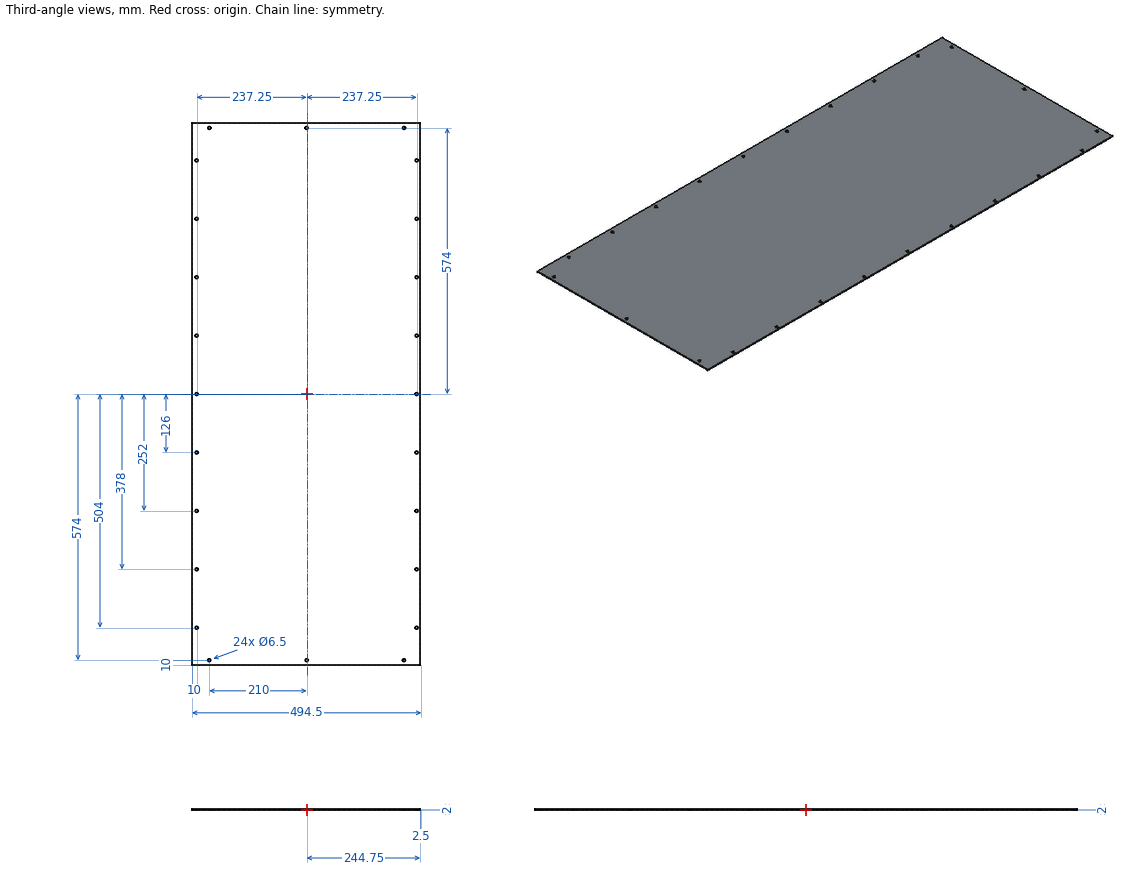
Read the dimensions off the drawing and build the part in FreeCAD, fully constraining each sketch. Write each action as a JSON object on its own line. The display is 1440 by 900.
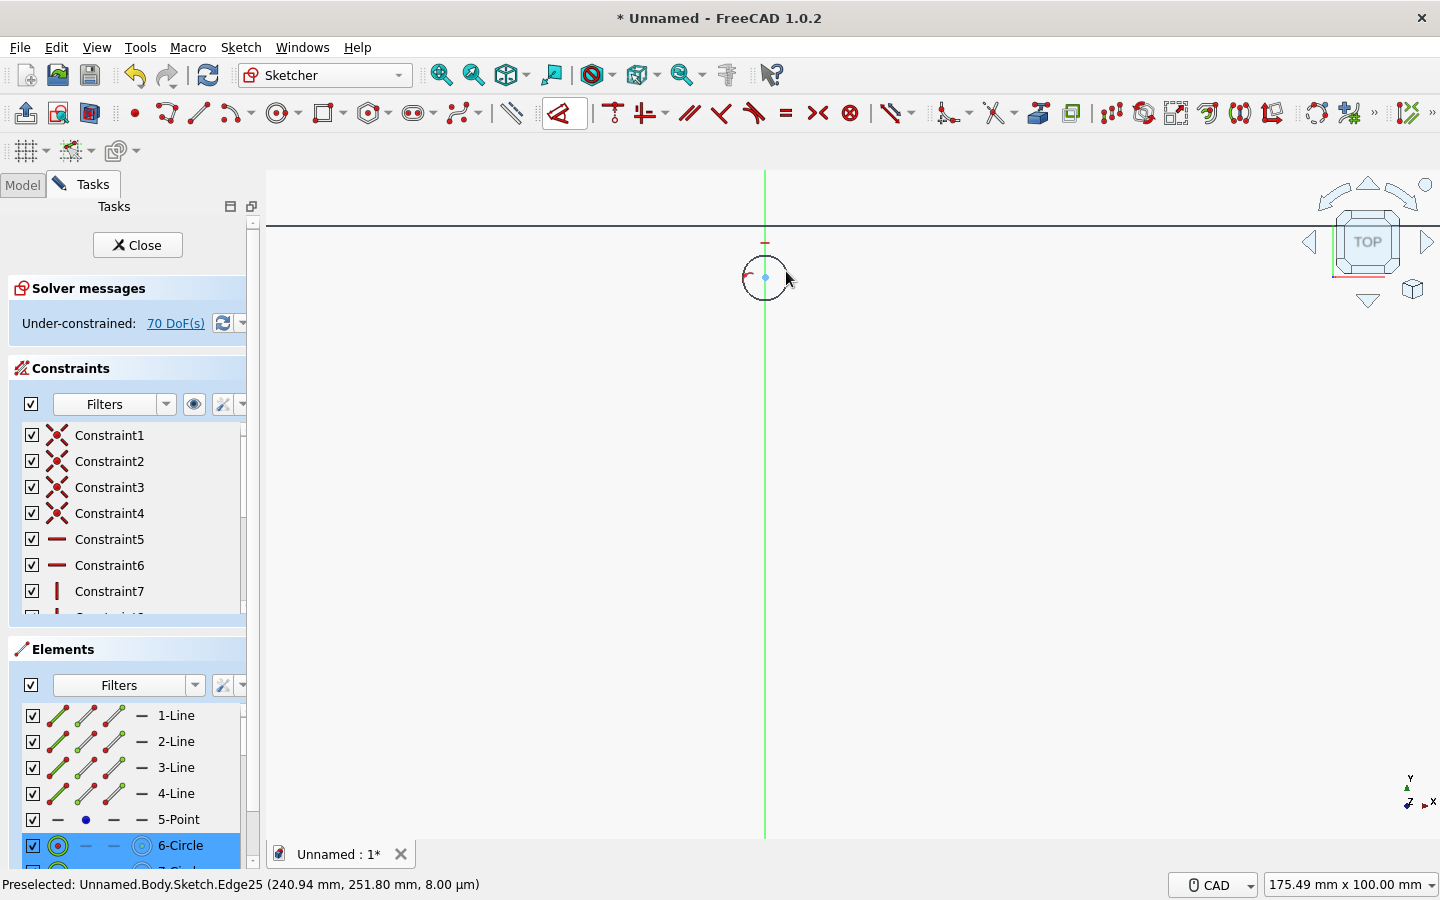
{"action": "left_click", "coordinate": [781, 262]}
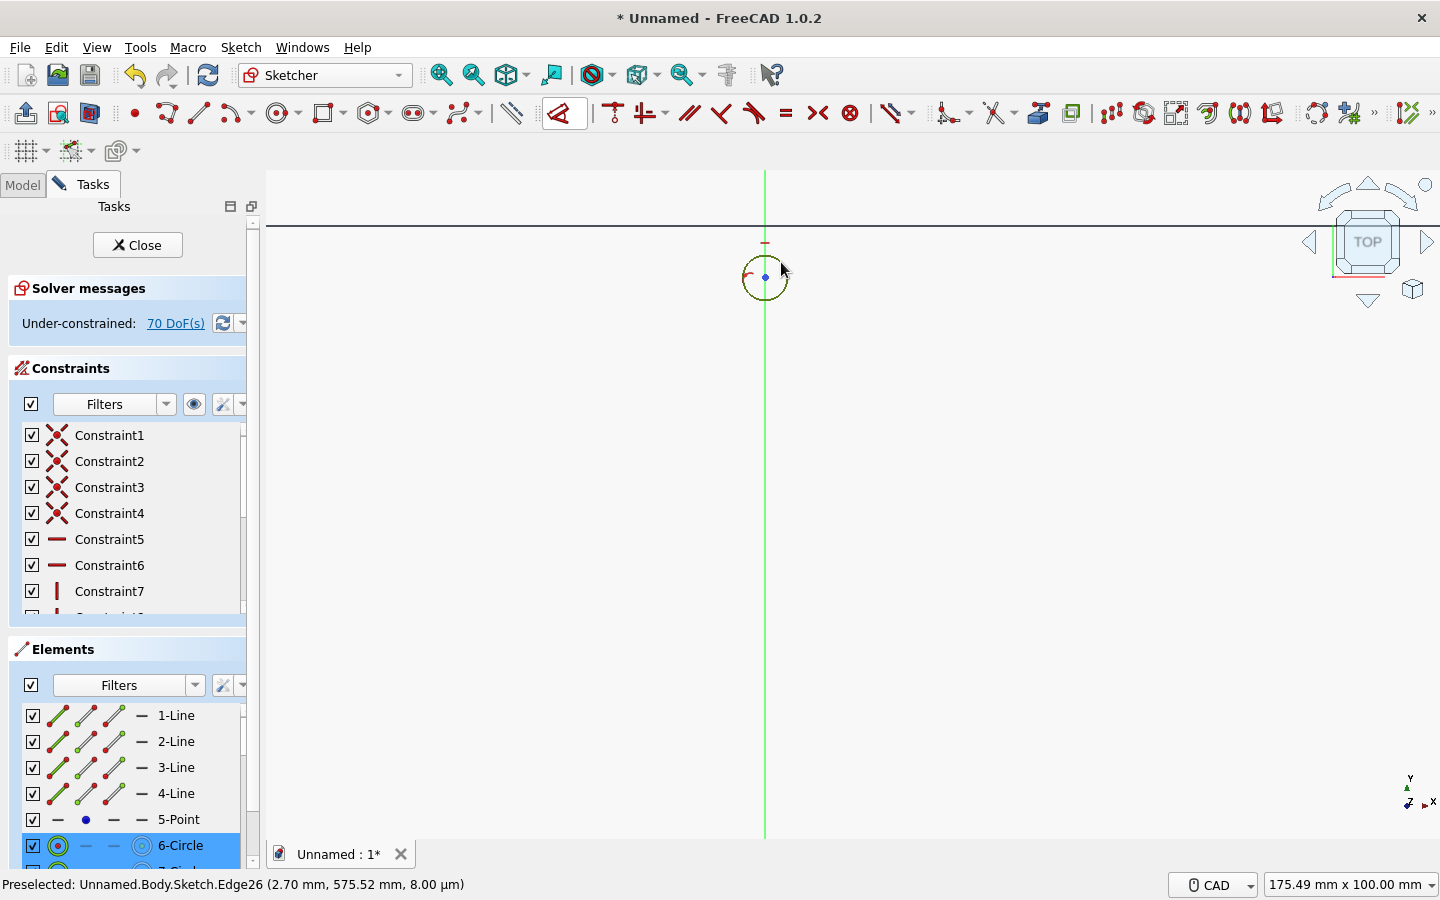
{"action": "scroll", "coordinate": [786, 271], "scroll_direction": "down", "scroll_amount": 14}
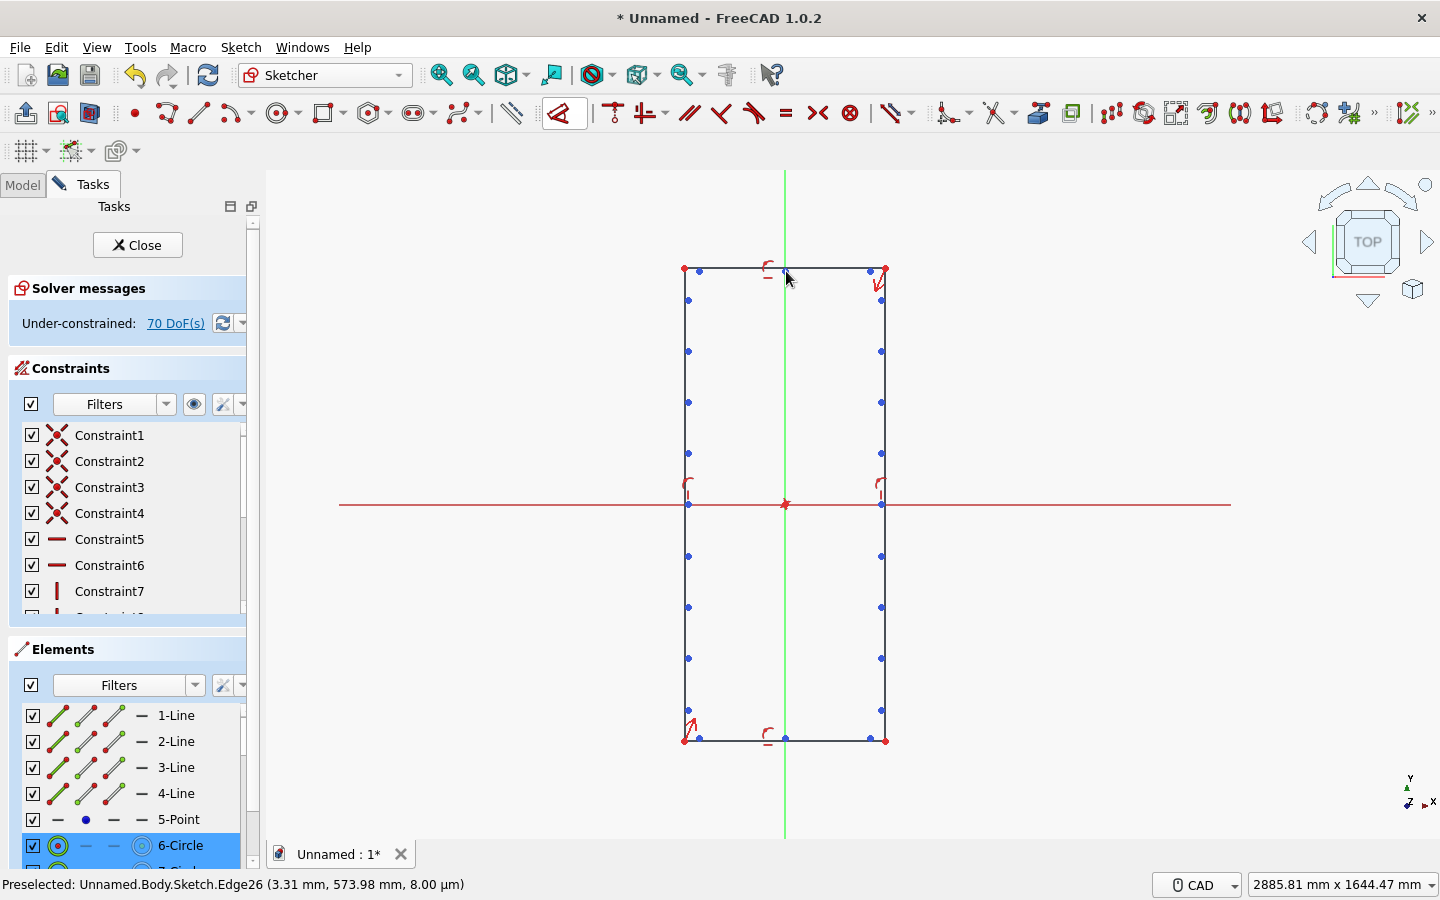
{"action": "scroll", "coordinate": [883, 350], "scroll_direction": "up", "scroll_amount": 12}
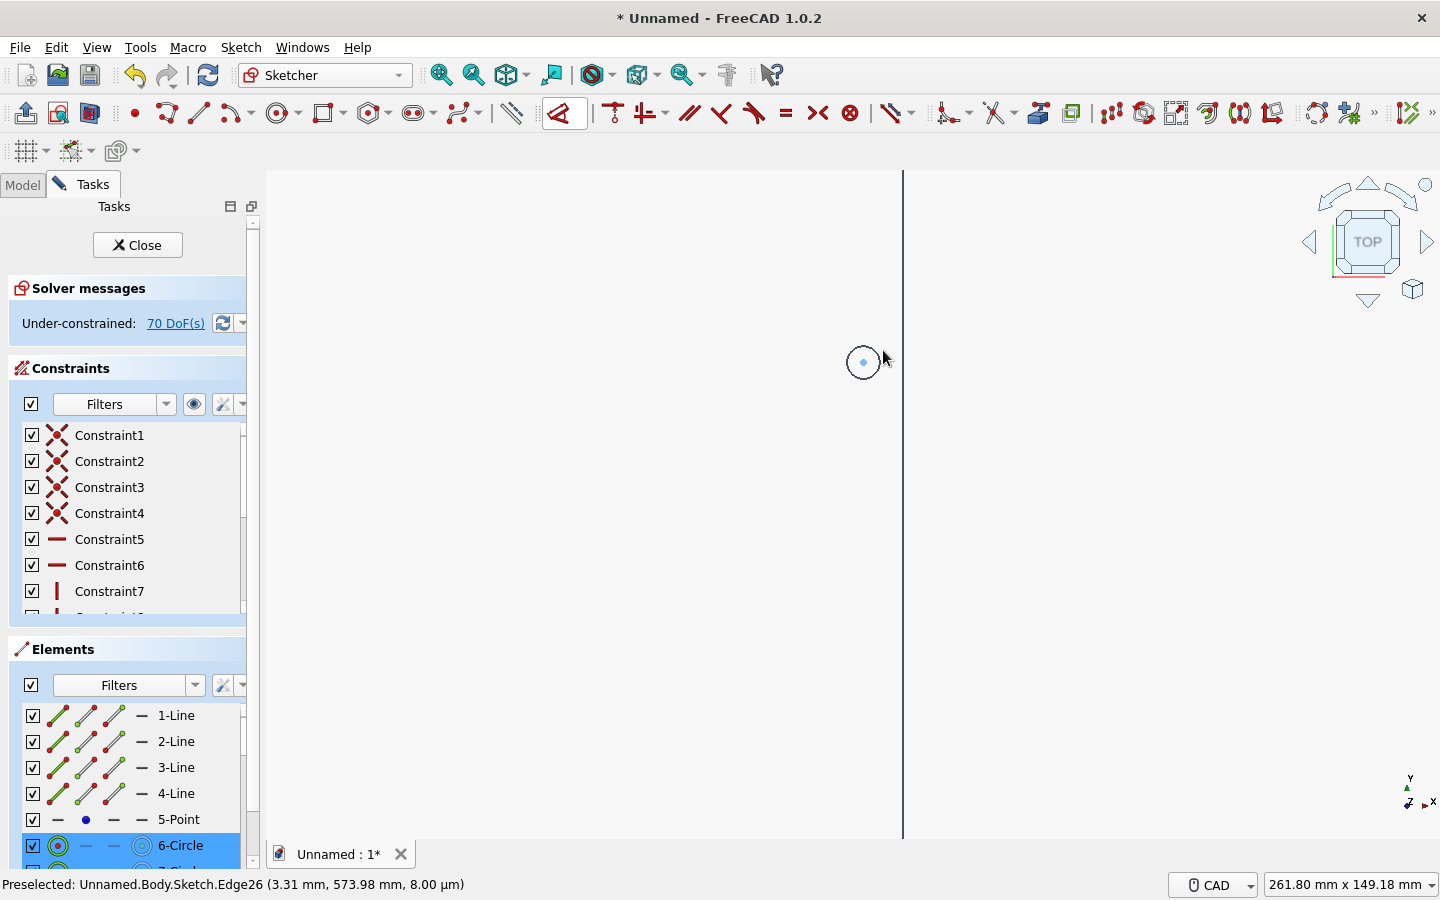
{"action": "left_click", "coordinate": [875, 351]}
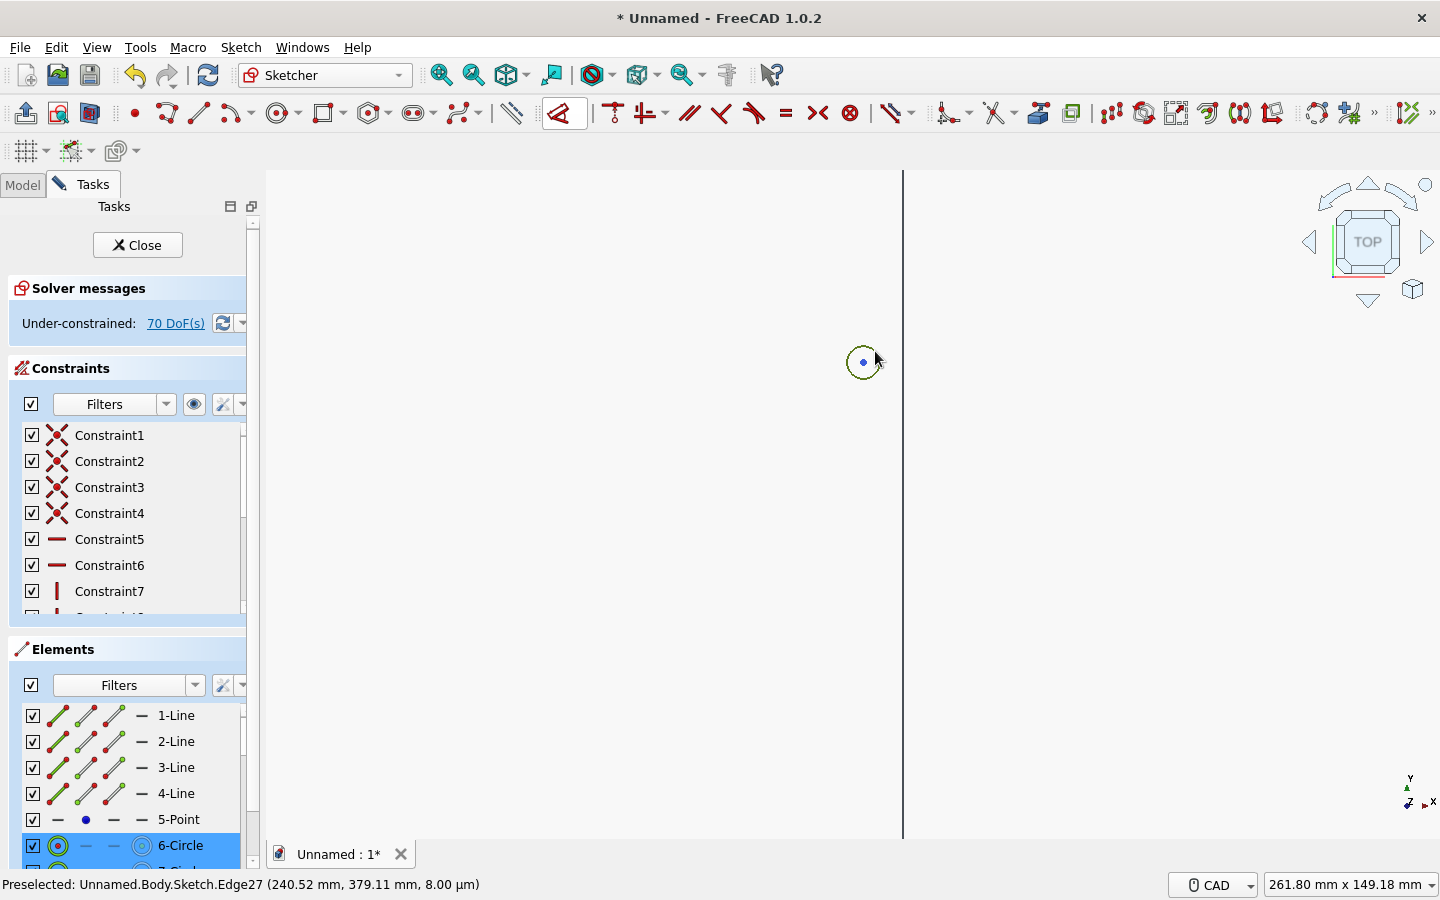
{"action": "scroll", "coordinate": [883, 350], "scroll_direction": "down", "scroll_amount": 12}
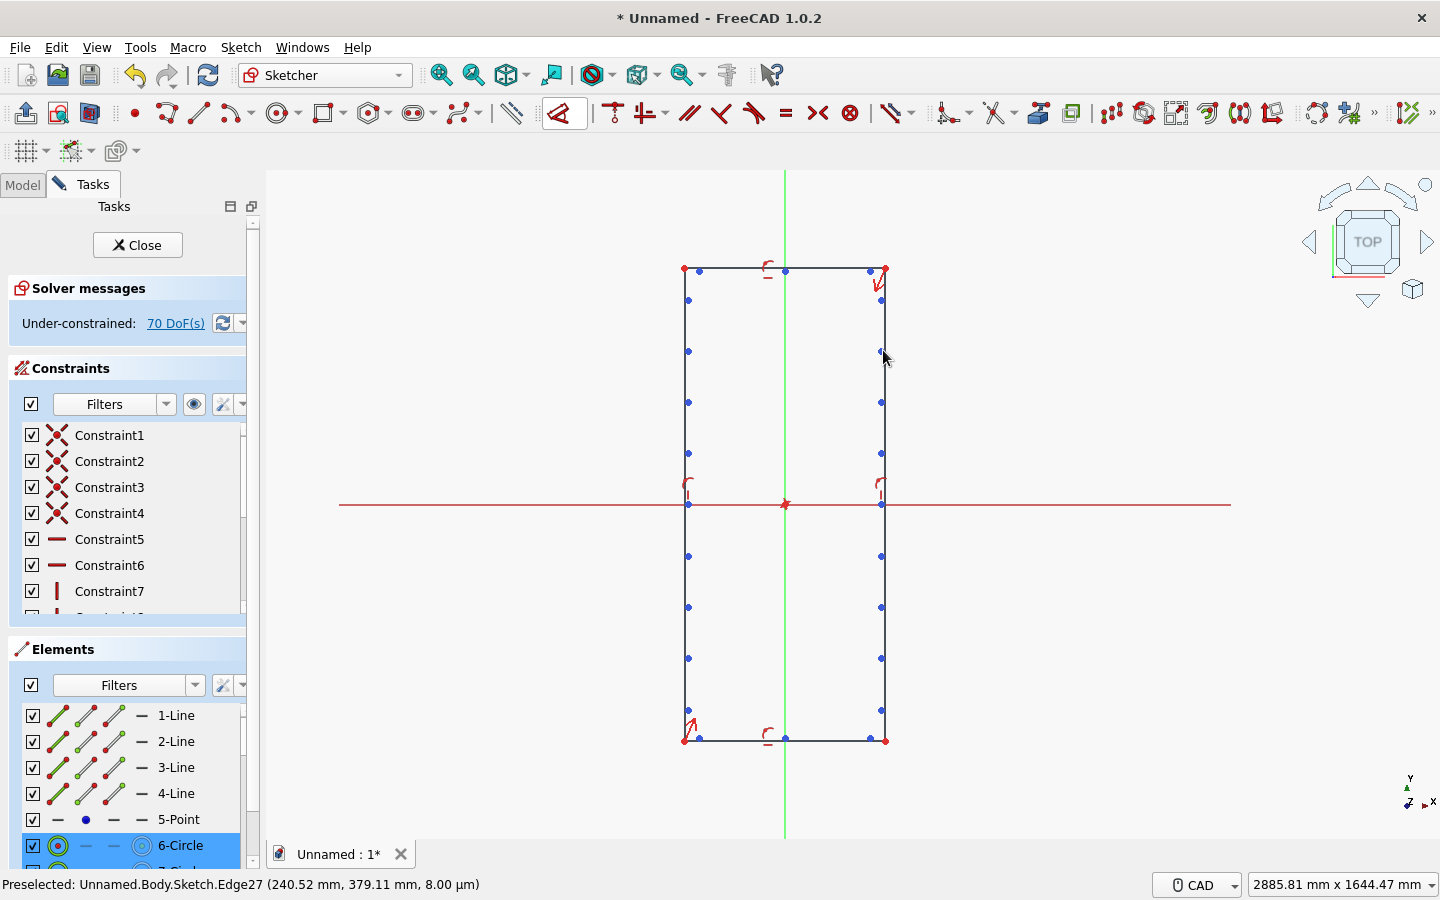
{"action": "scroll", "coordinate": [883, 299], "scroll_direction": "up", "scroll_amount": 12}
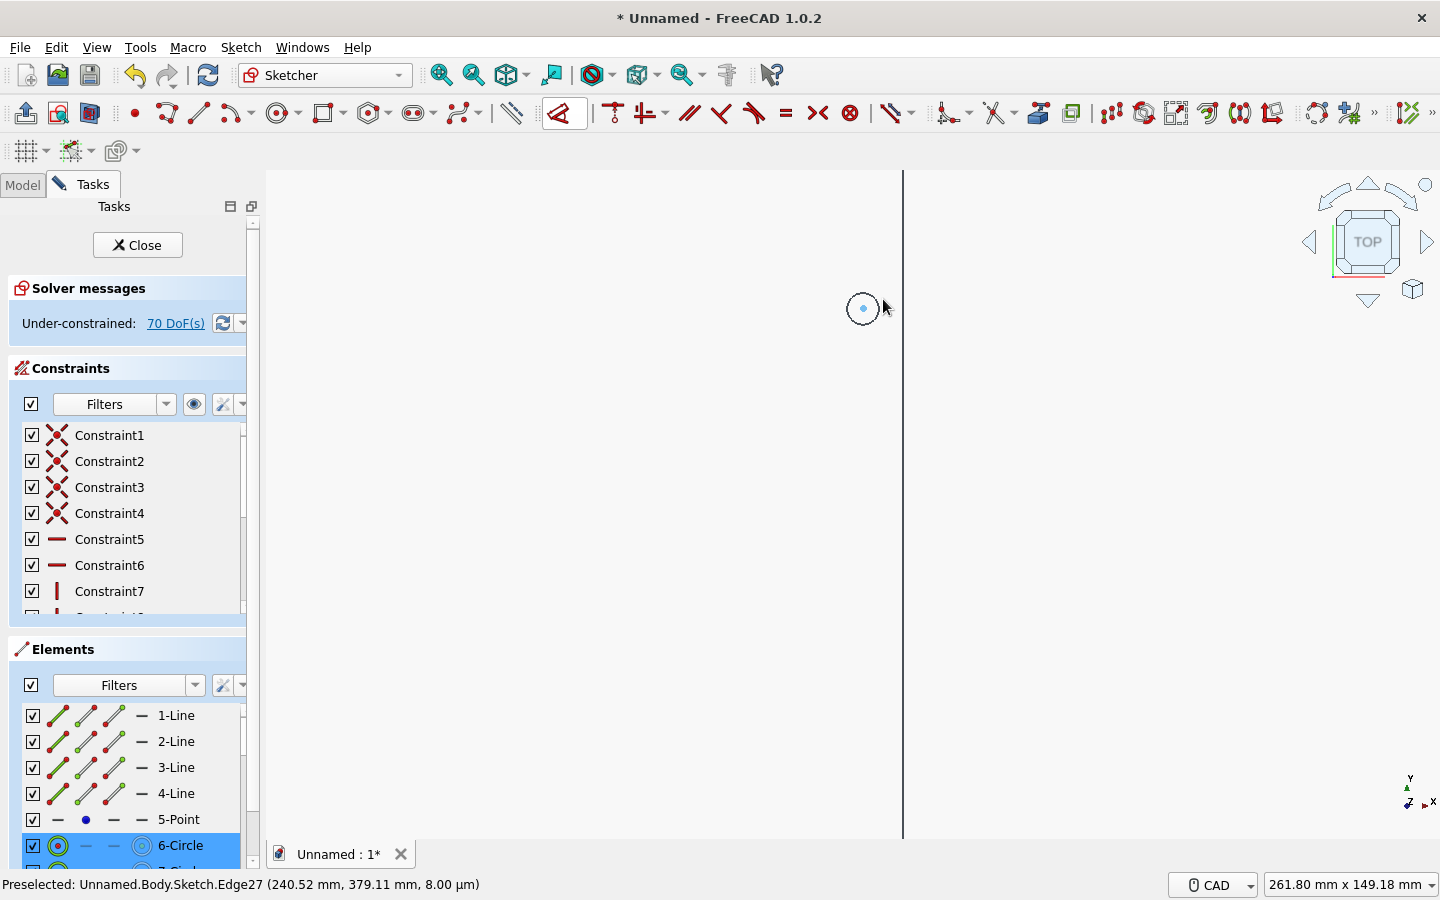
{"action": "left_click", "coordinate": [874, 298]}